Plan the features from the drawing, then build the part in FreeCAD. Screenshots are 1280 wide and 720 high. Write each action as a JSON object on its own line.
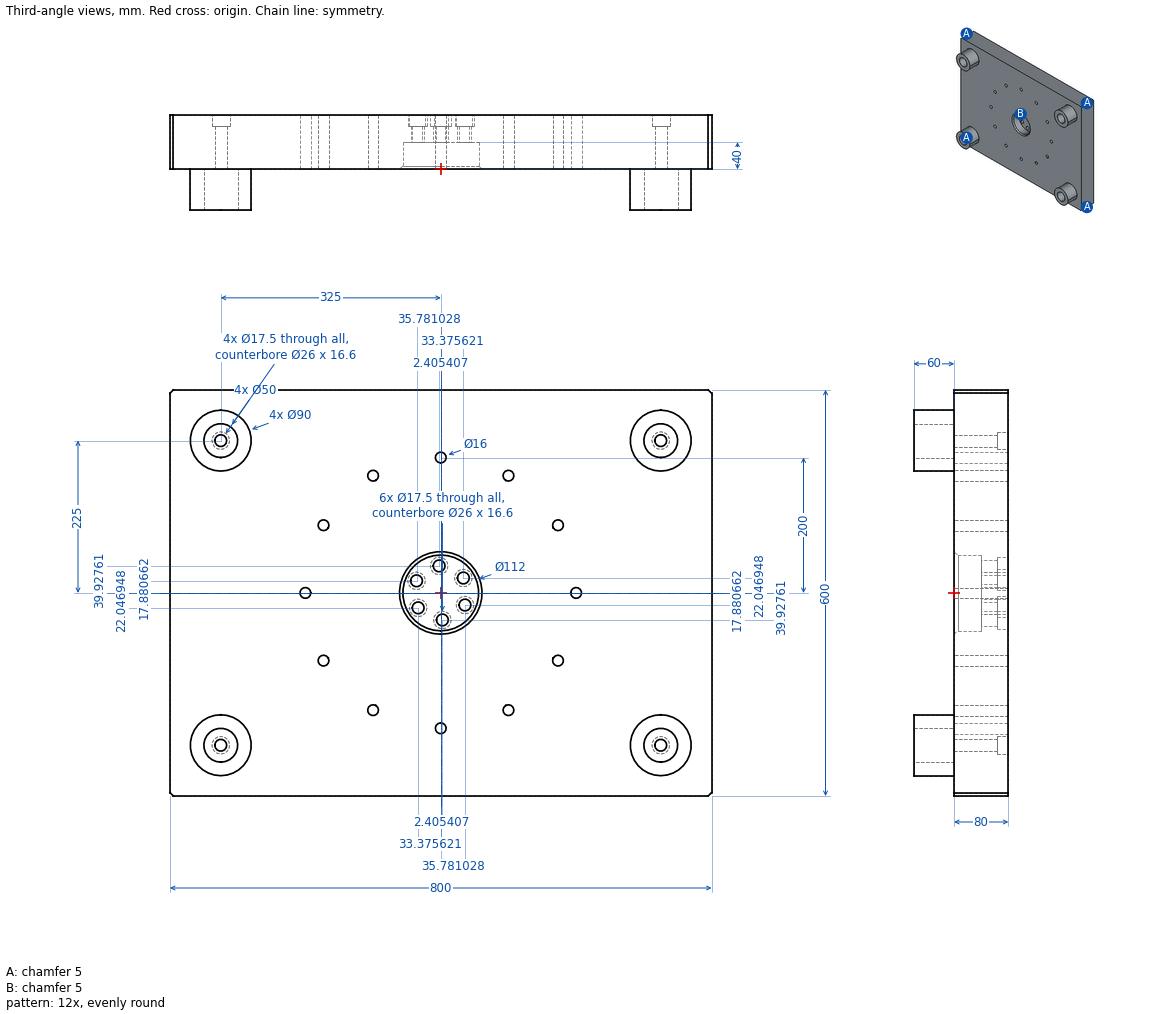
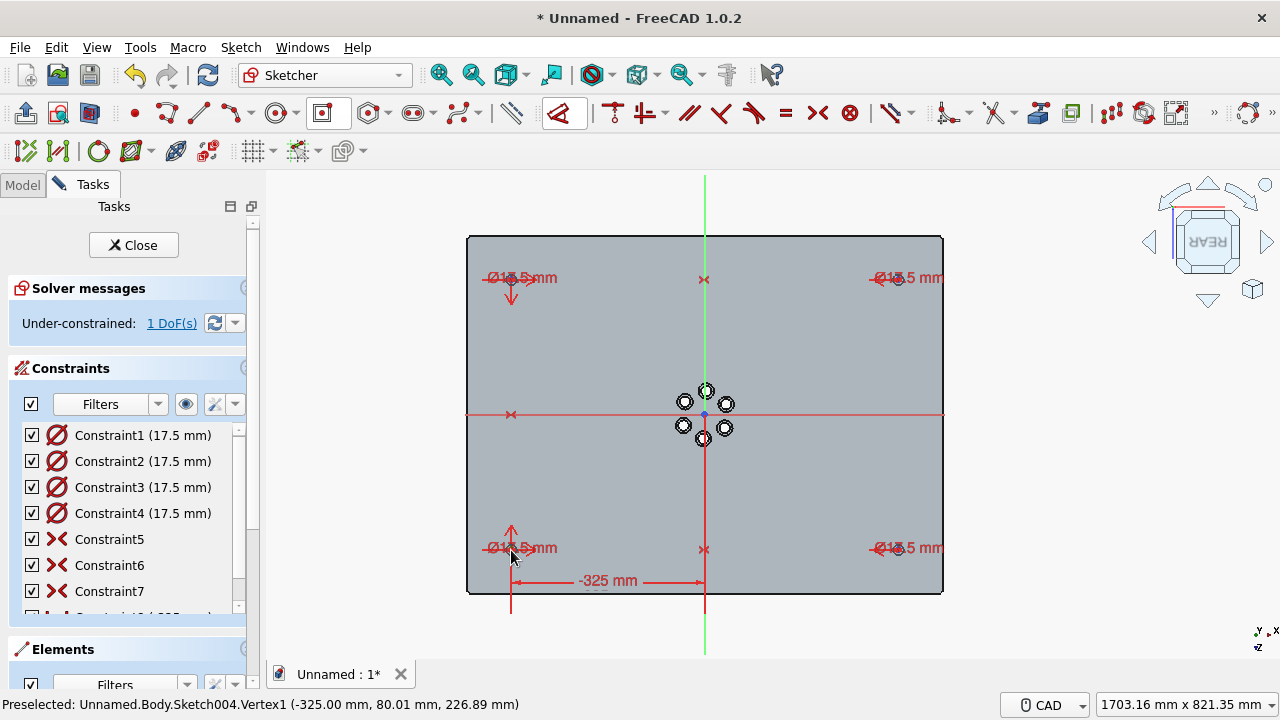
{"action": "key", "text": "i"}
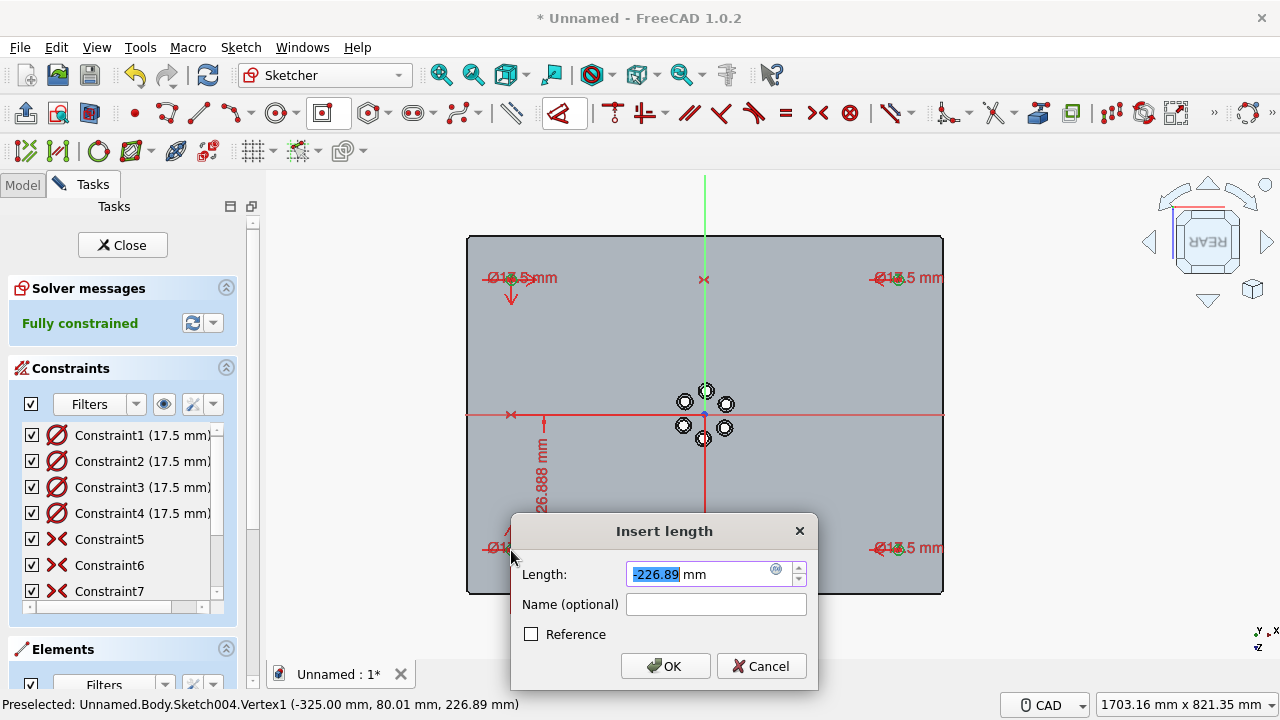
{"action": "type", "text": "-225"}
{"action": "key", "text": "Return"}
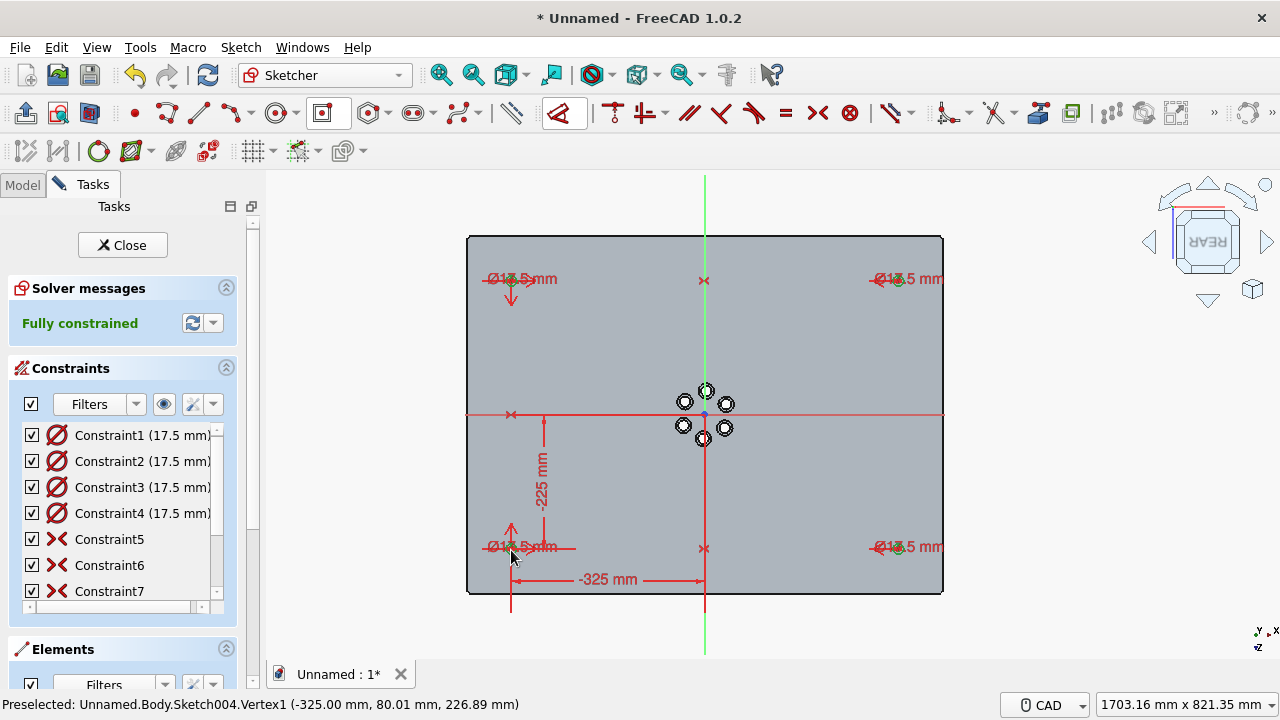
{"action": "left_click", "coordinate": [123, 245]}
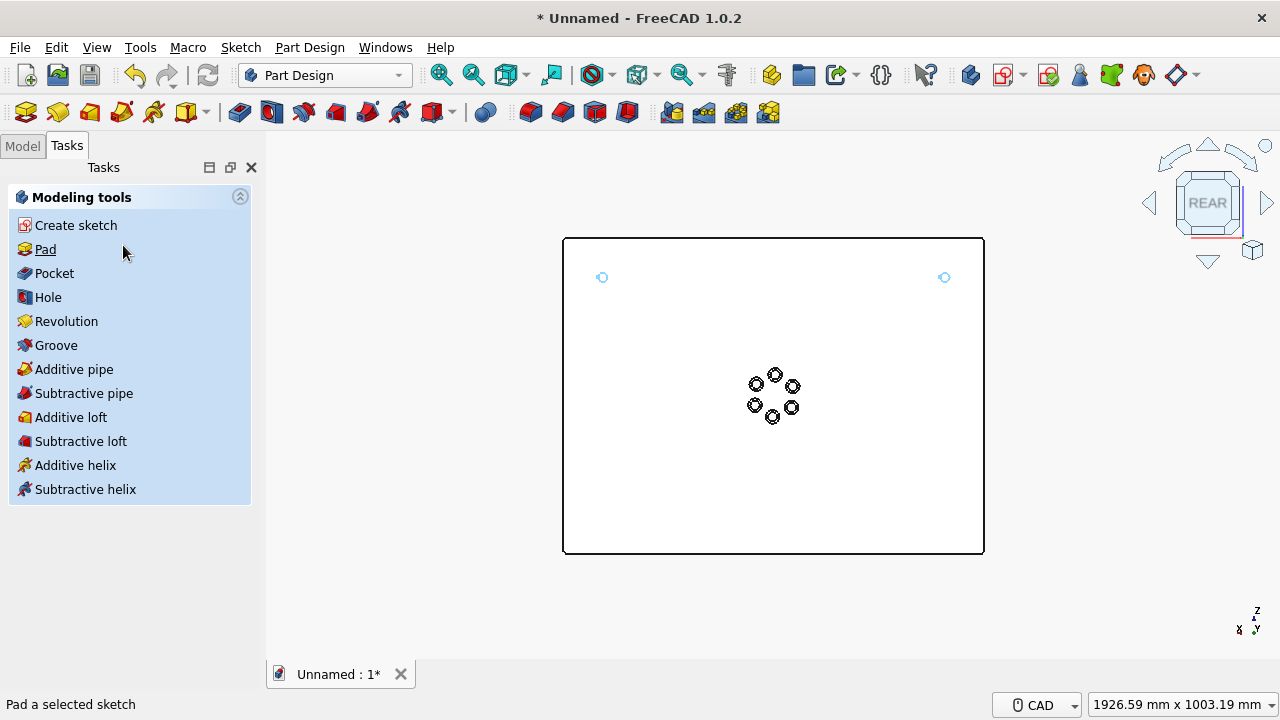
{"action": "left_click", "coordinate": [272, 112]}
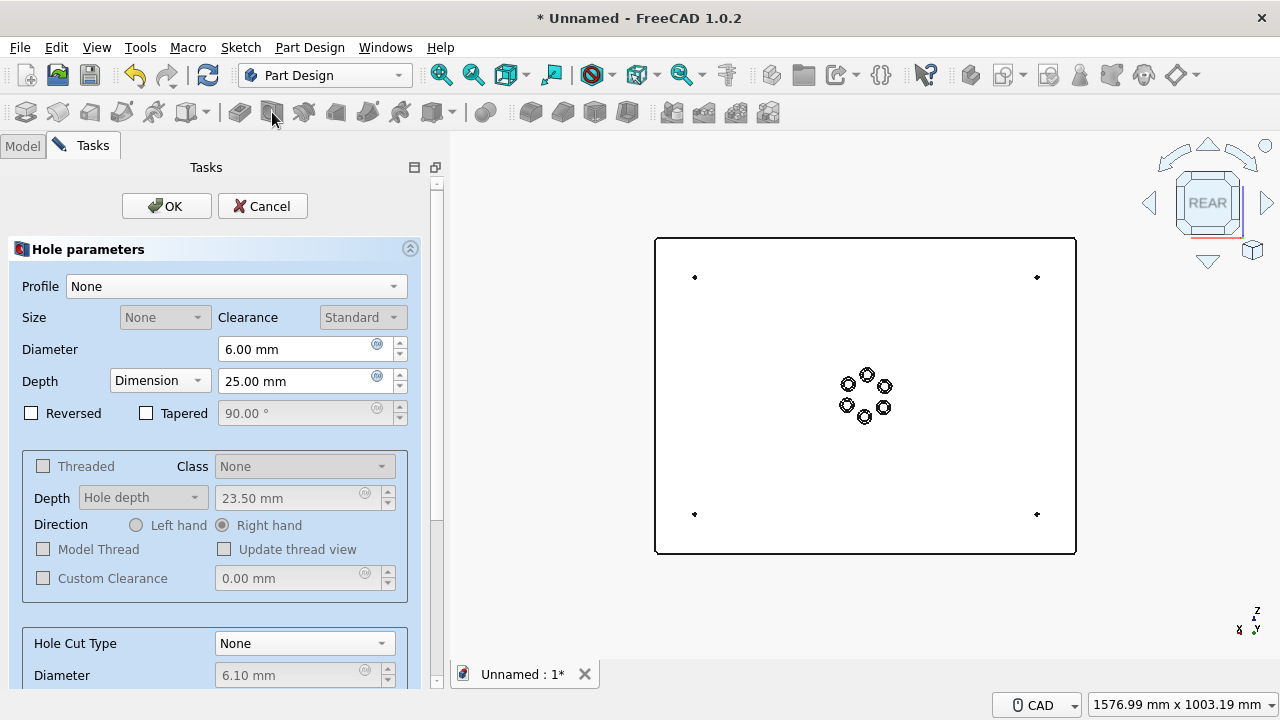
{"action": "triple_click", "coordinate": [305, 349]}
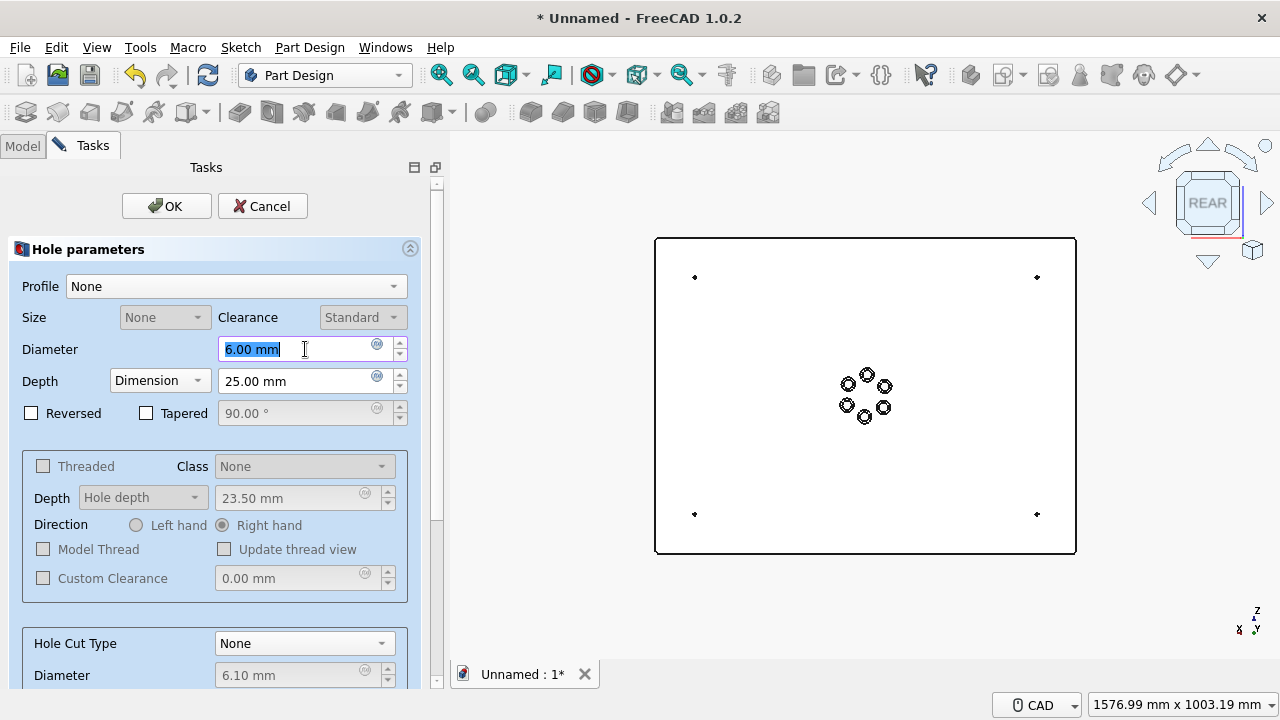
{"action": "type", "text": "17.5"}
{"action": "key", "text": "Tab"}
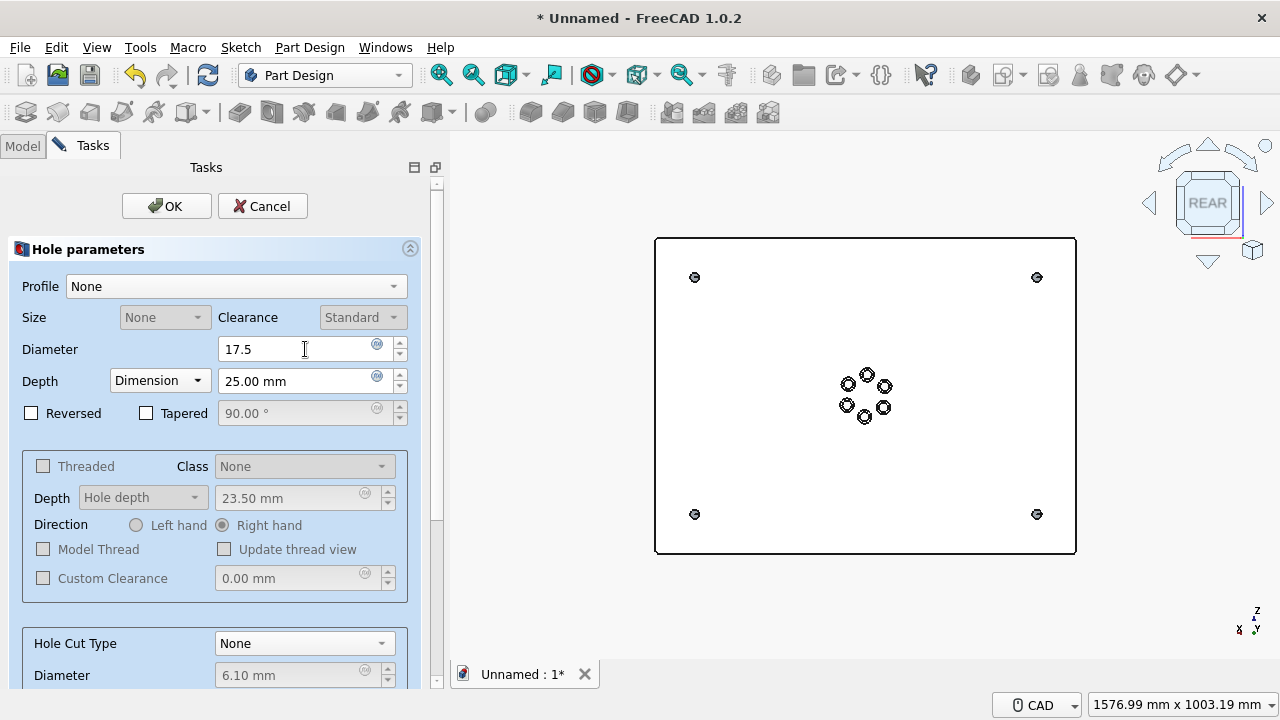
{"action": "left_click", "coordinate": [161, 380]}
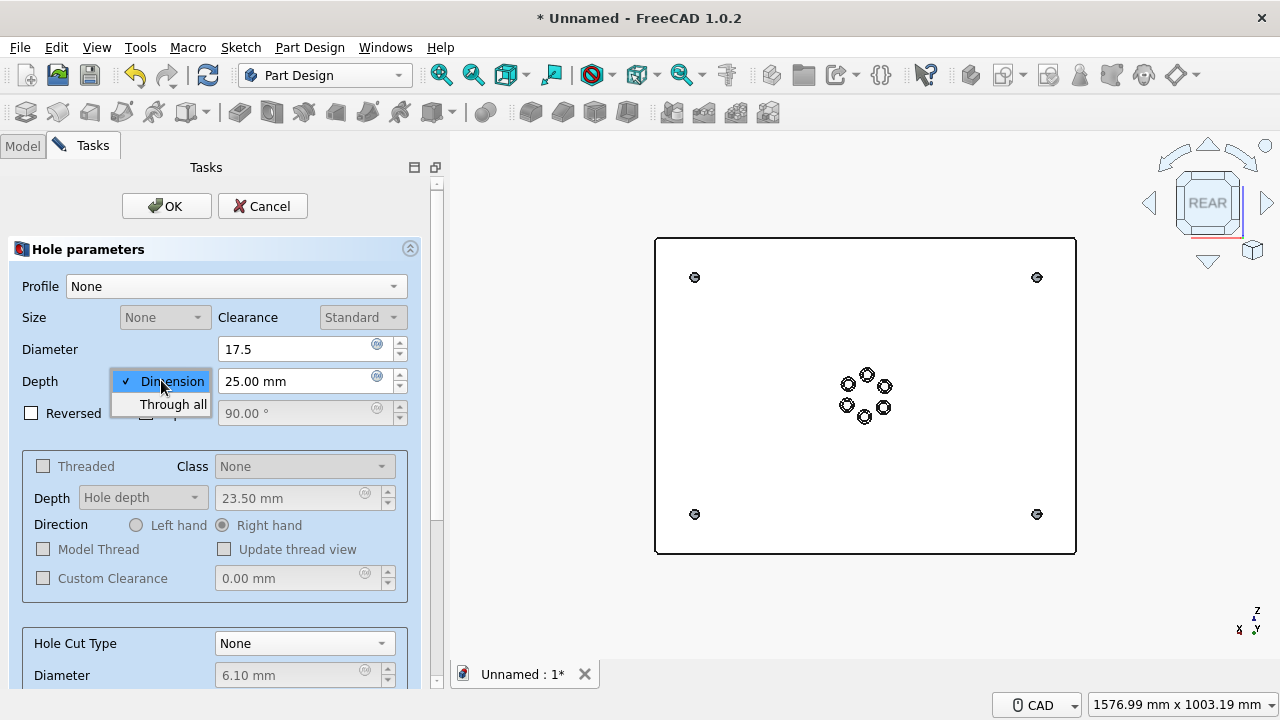
{"action": "left_click", "coordinate": [160, 404]}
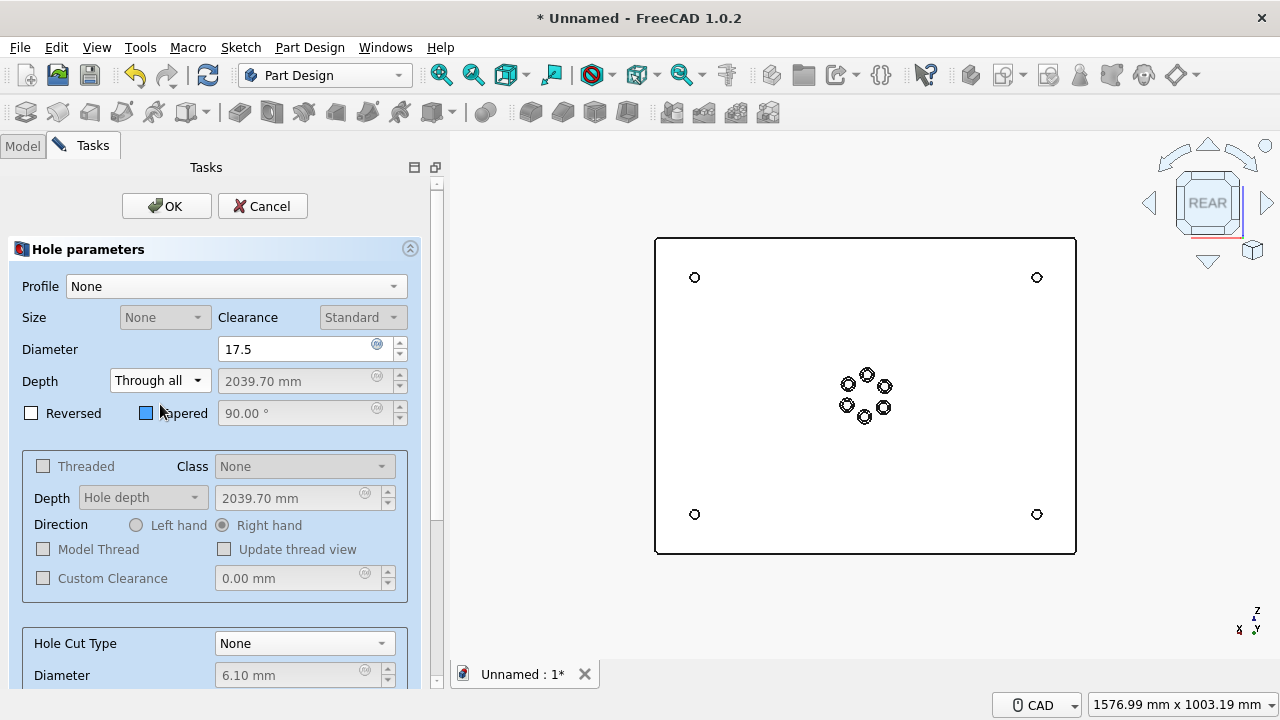
{"action": "left_click", "coordinate": [306, 644]}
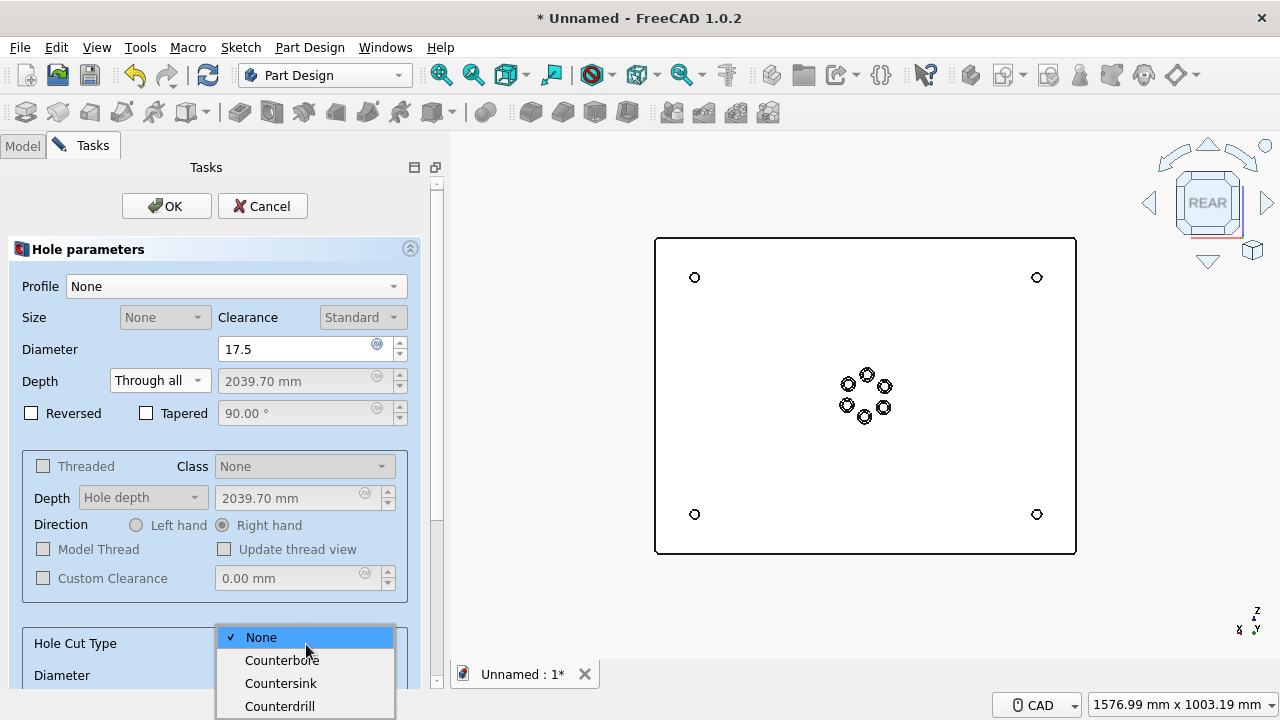
{"action": "left_click", "coordinate": [304, 660]}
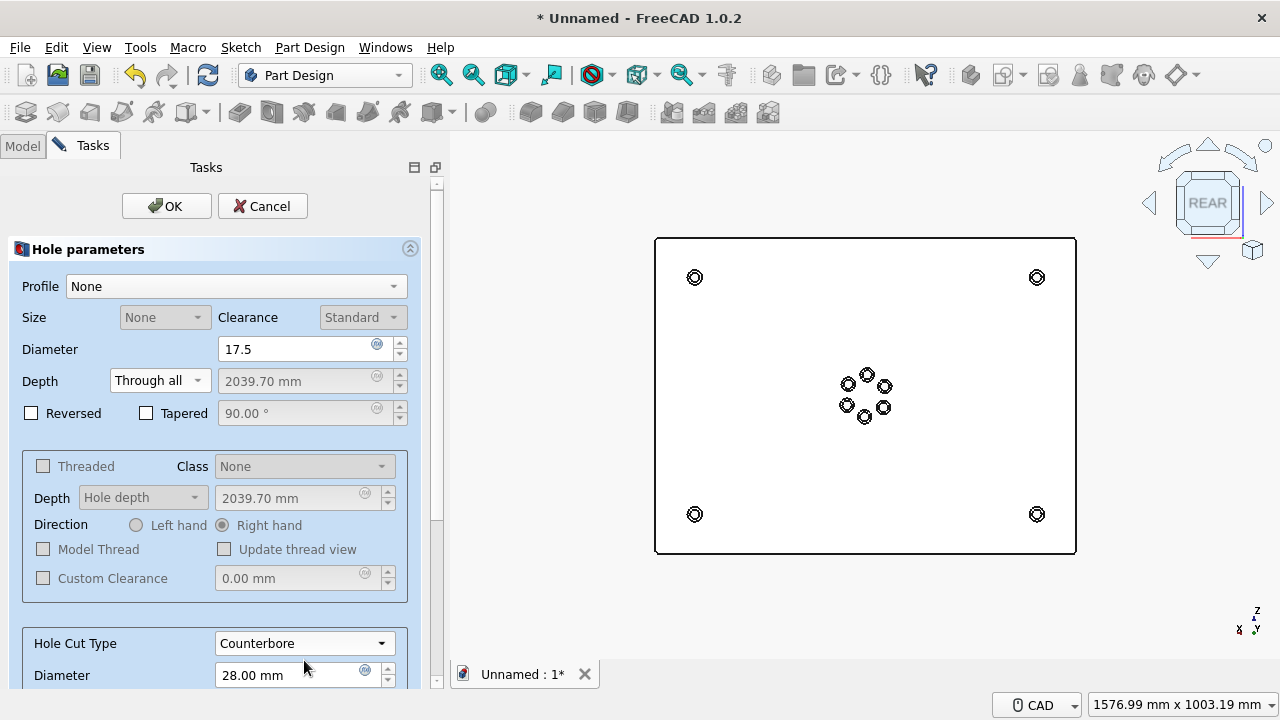
{"action": "triple_click", "coordinate": [298, 675]}